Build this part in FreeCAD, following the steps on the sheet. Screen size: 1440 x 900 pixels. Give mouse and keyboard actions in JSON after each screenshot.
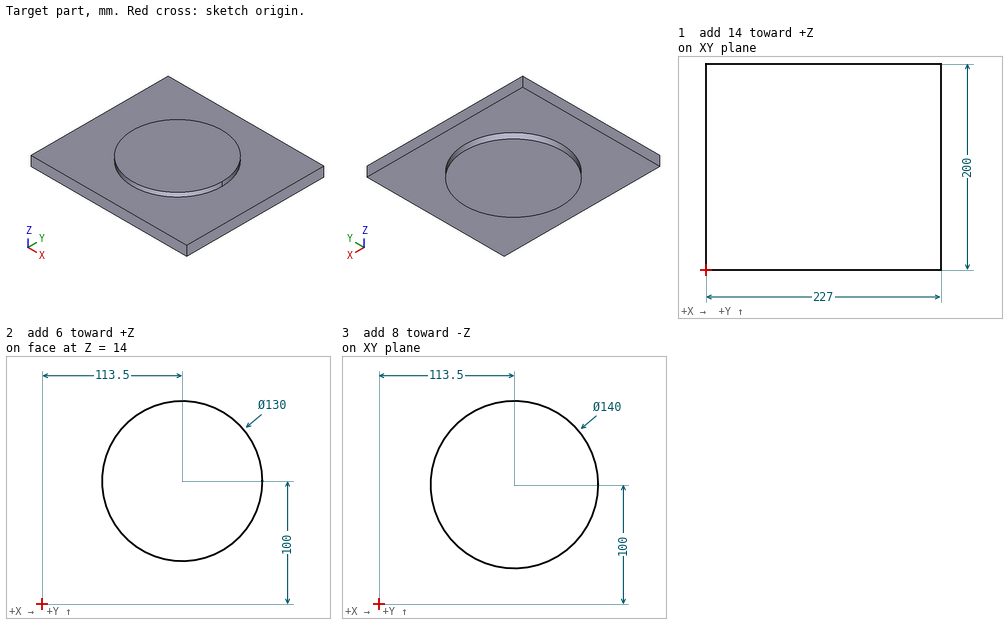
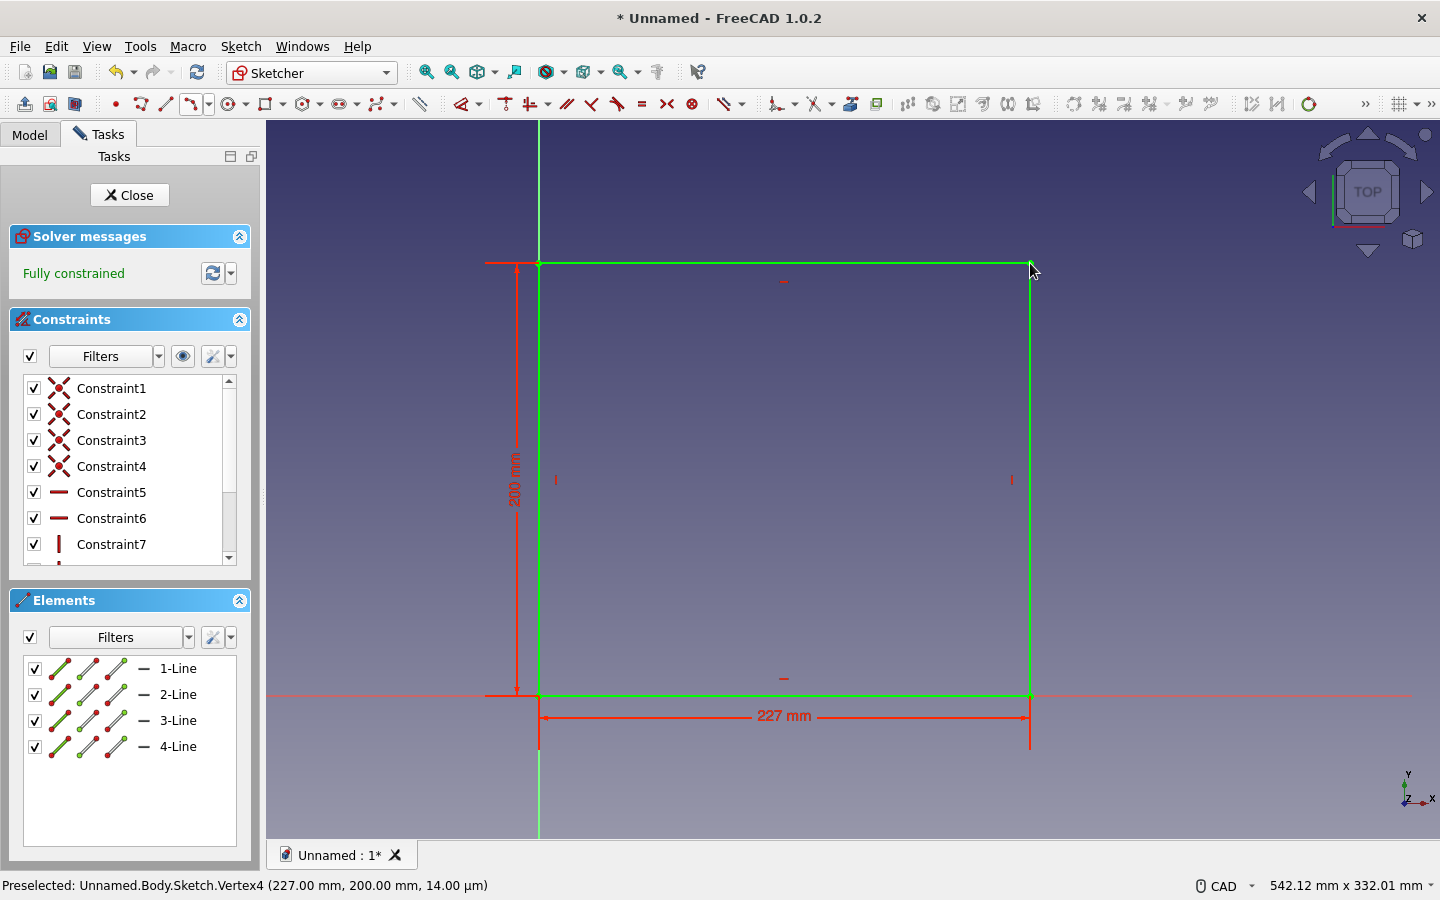
{"action": "left_click", "coordinate": [130, 195]}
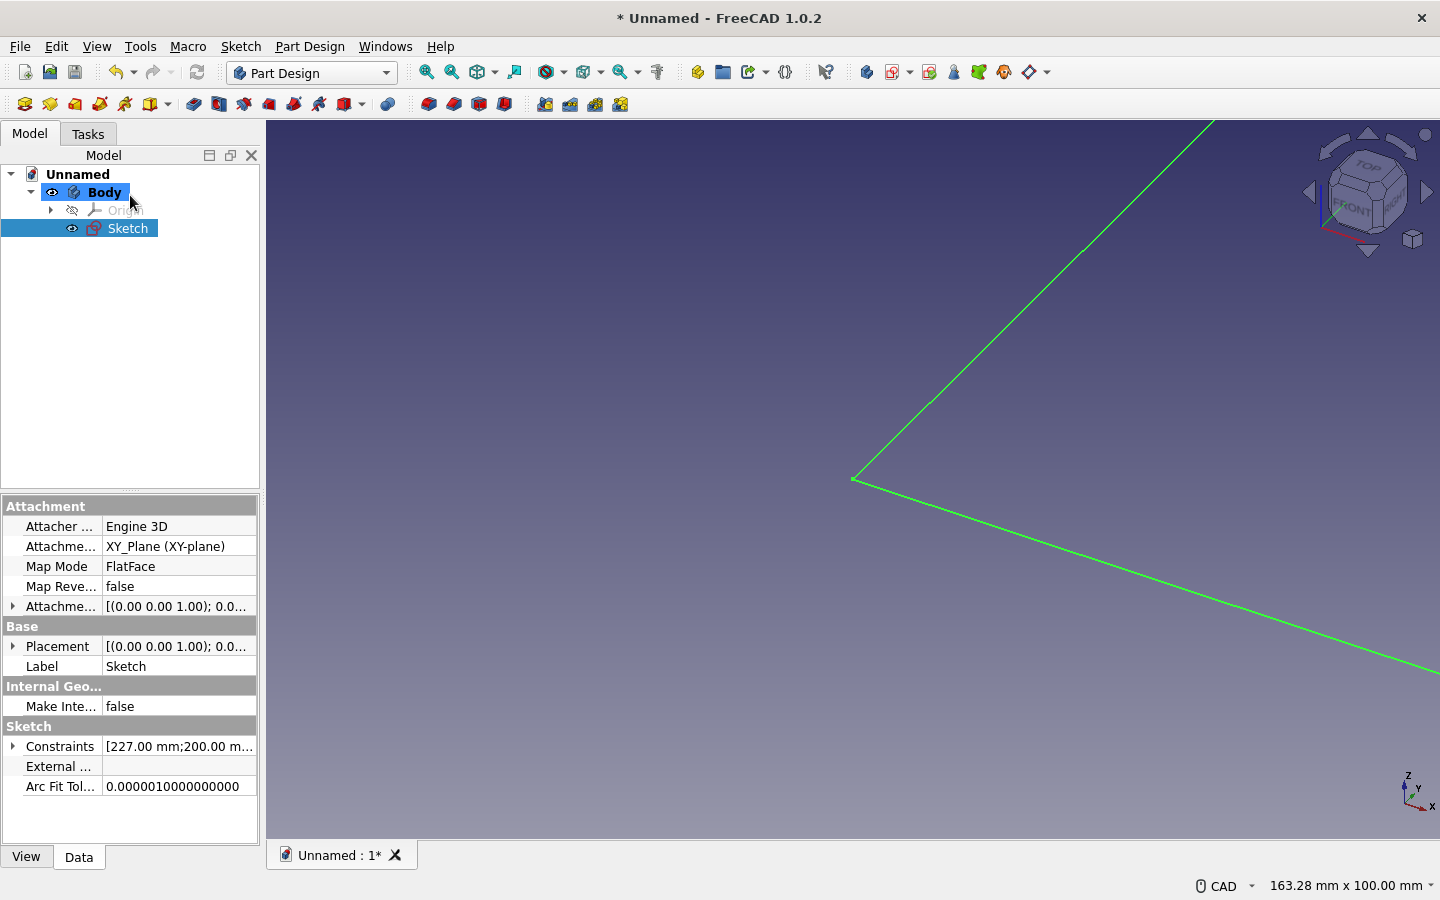
{"action": "left_click", "coordinate": [25, 104]}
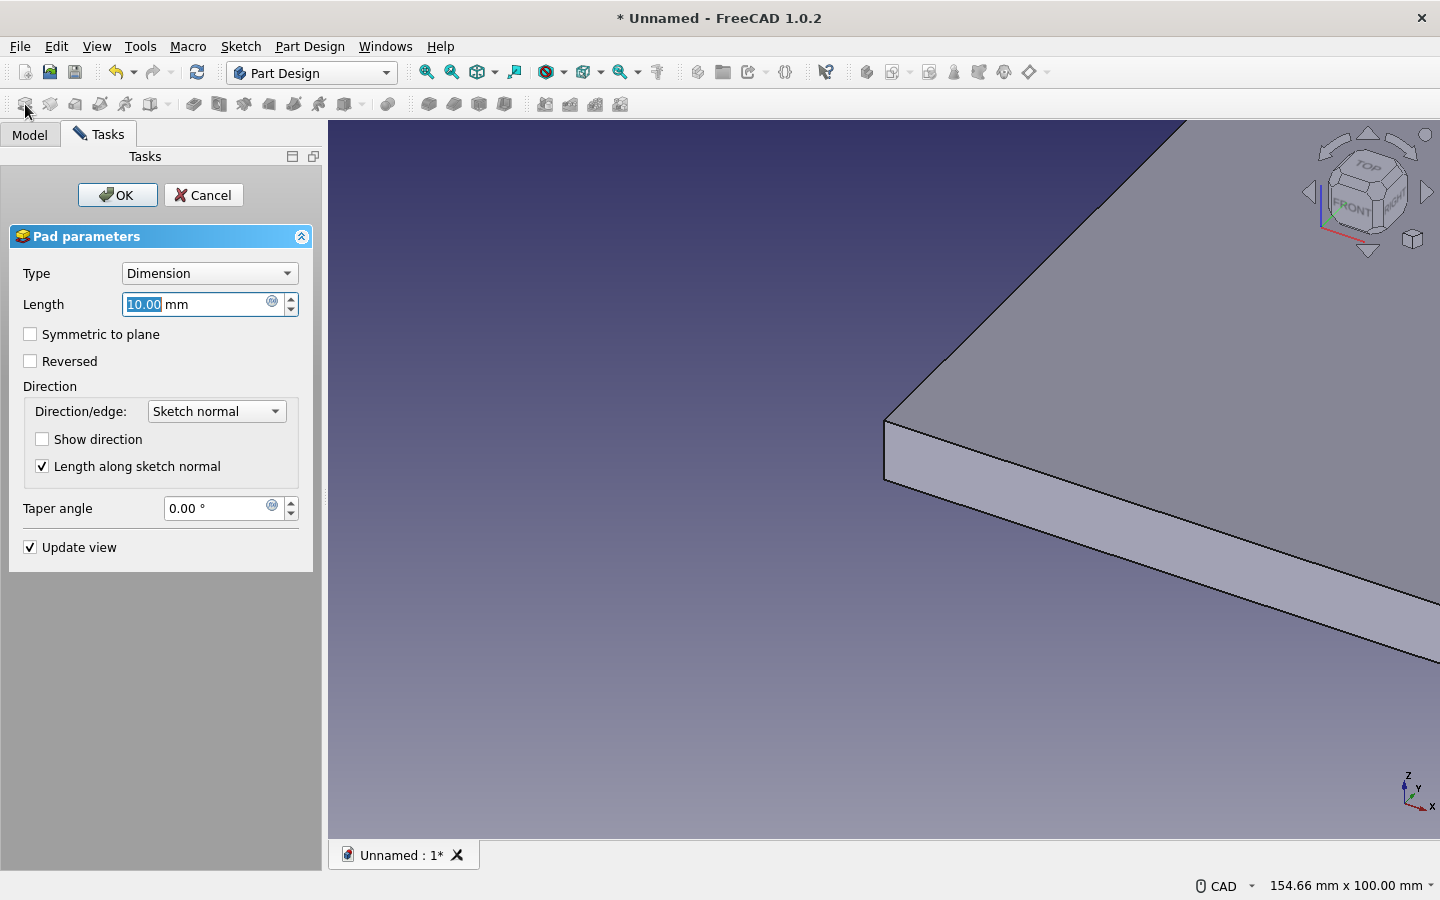
{"action": "type", "text": "14"}
{"action": "key", "text": "Tab"}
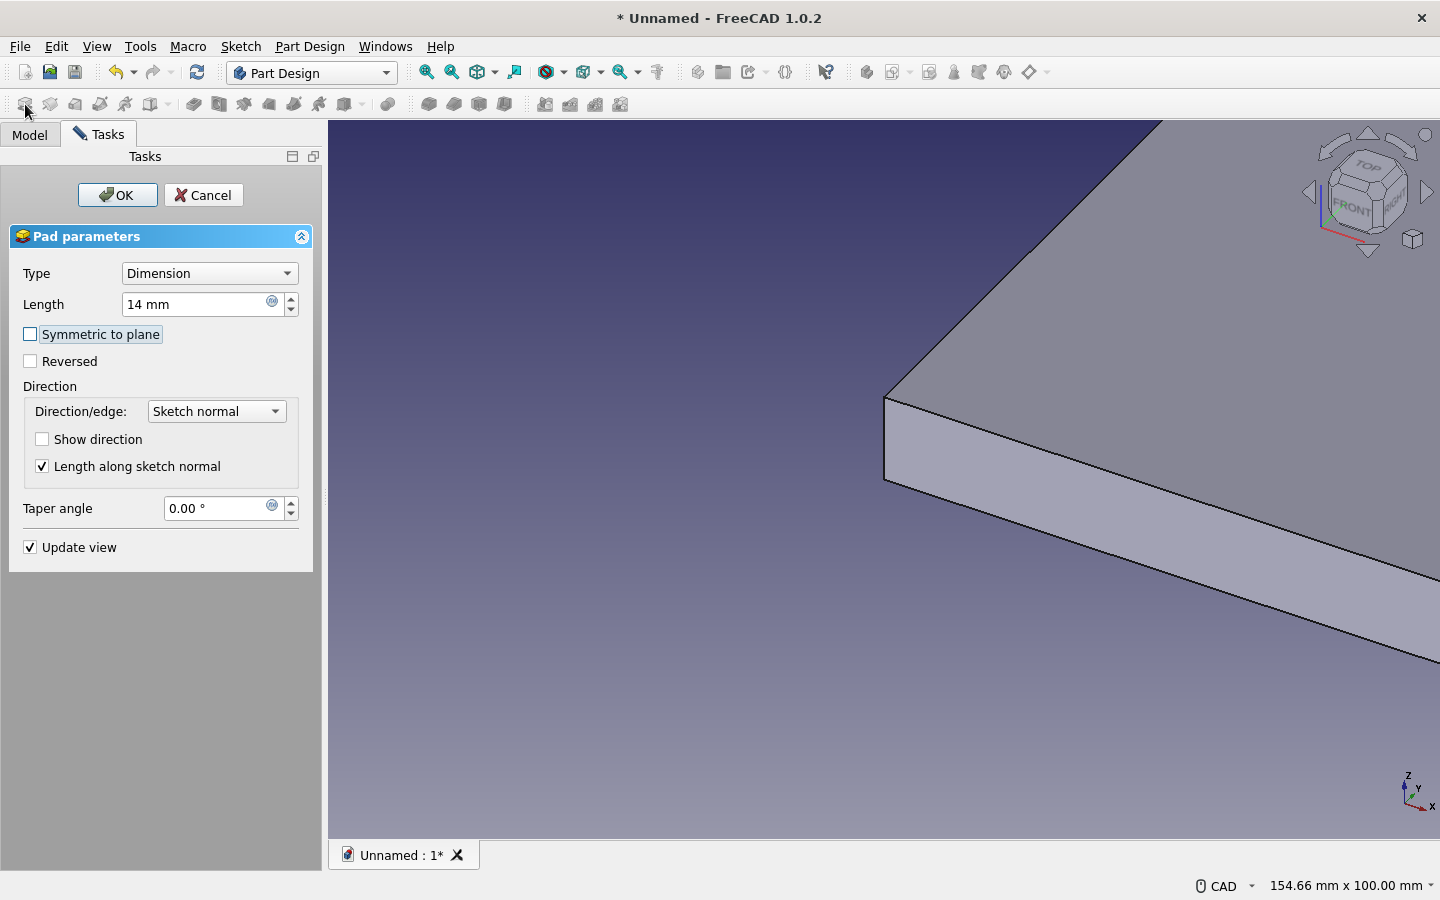
{"action": "left_click", "coordinate": [118, 195]}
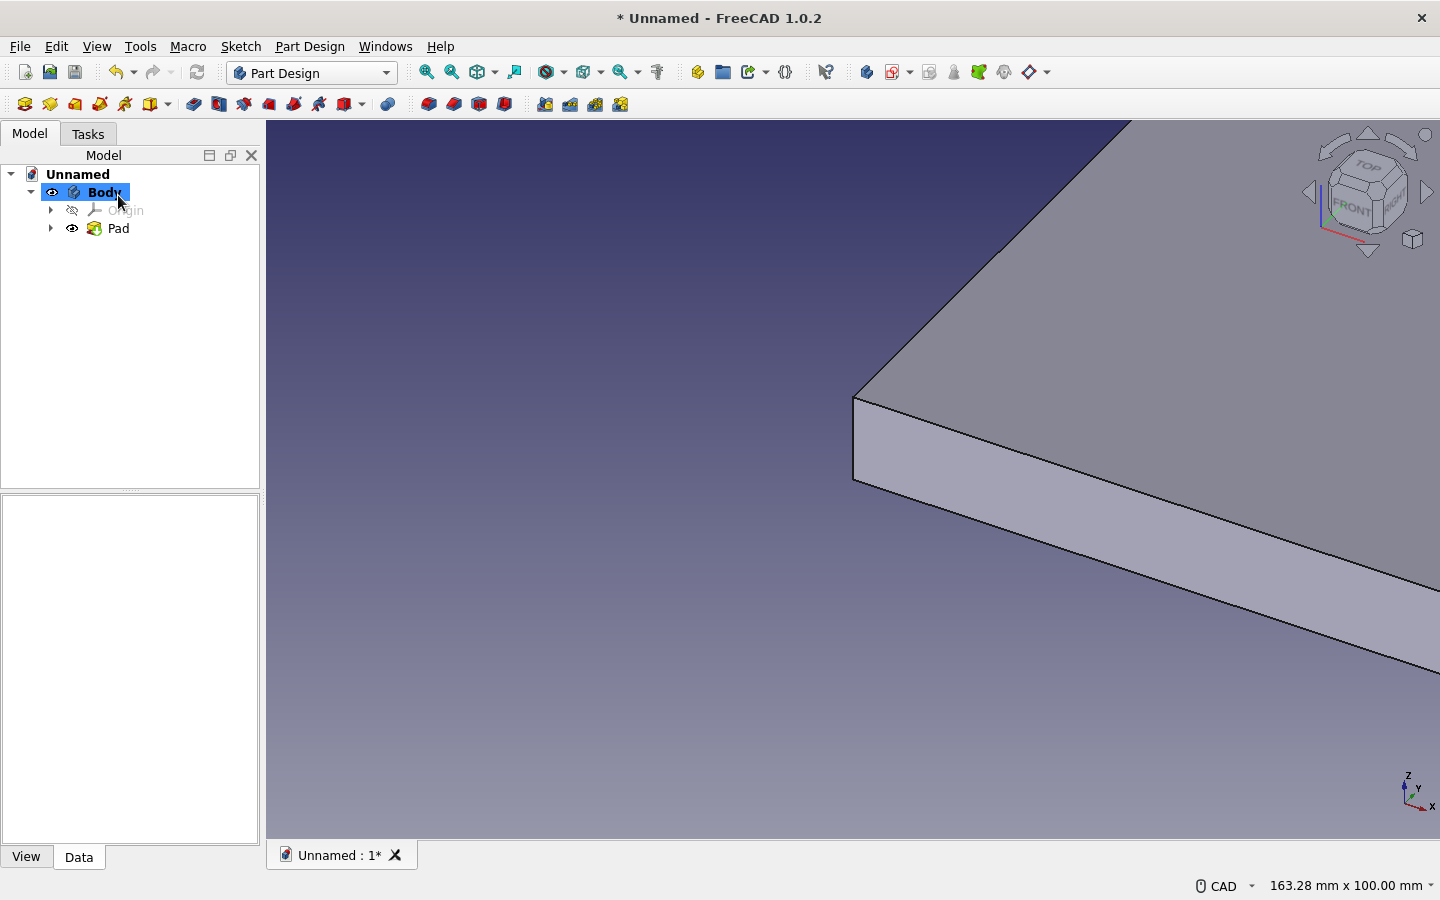
{"action": "left_click", "coordinate": [427, 72]}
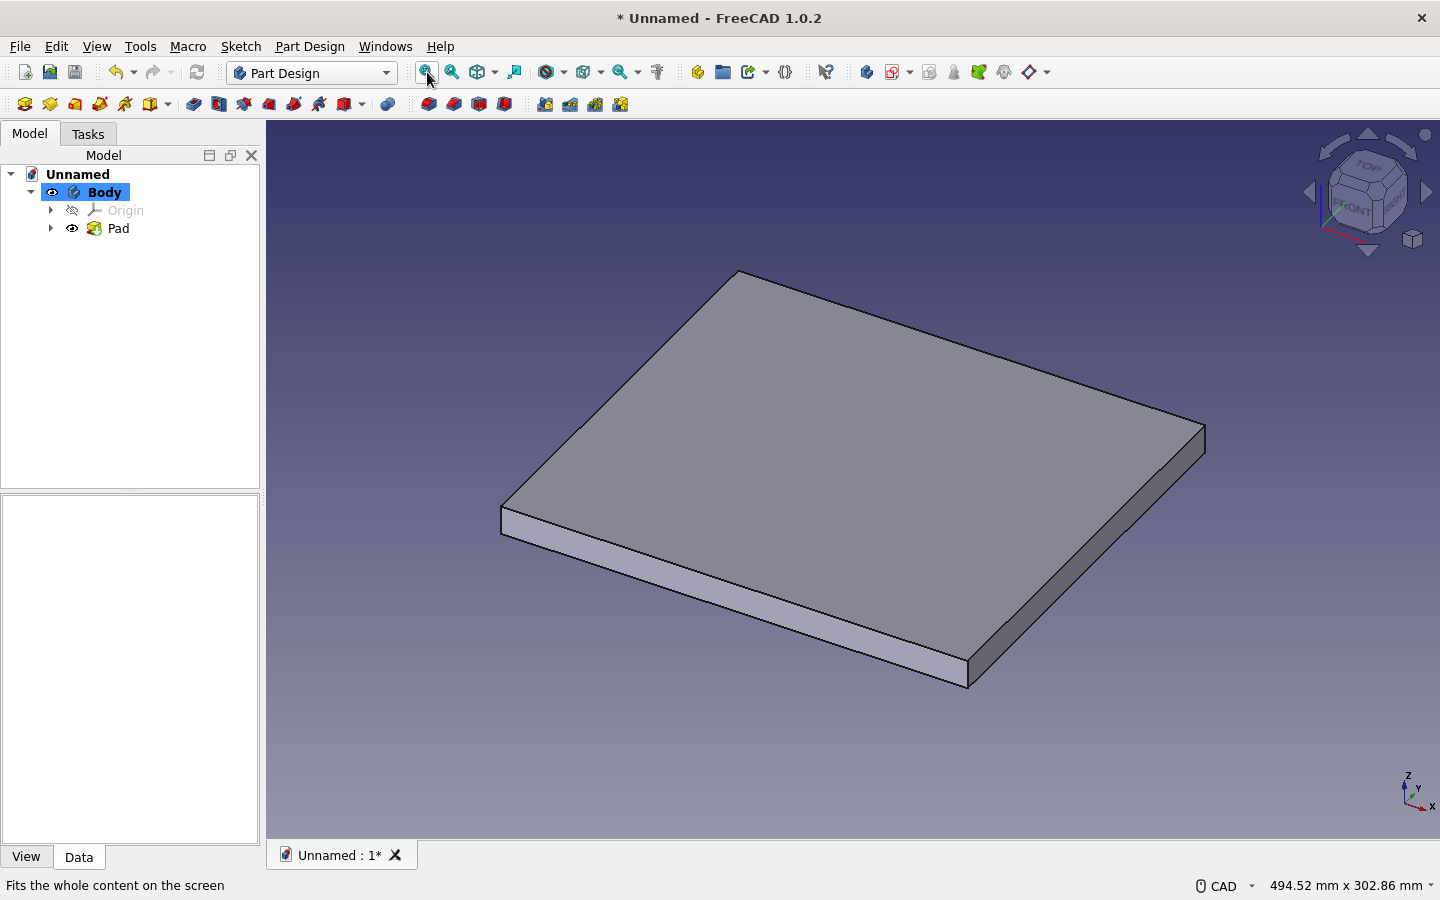
{"action": "left_click", "coordinate": [853, 465]}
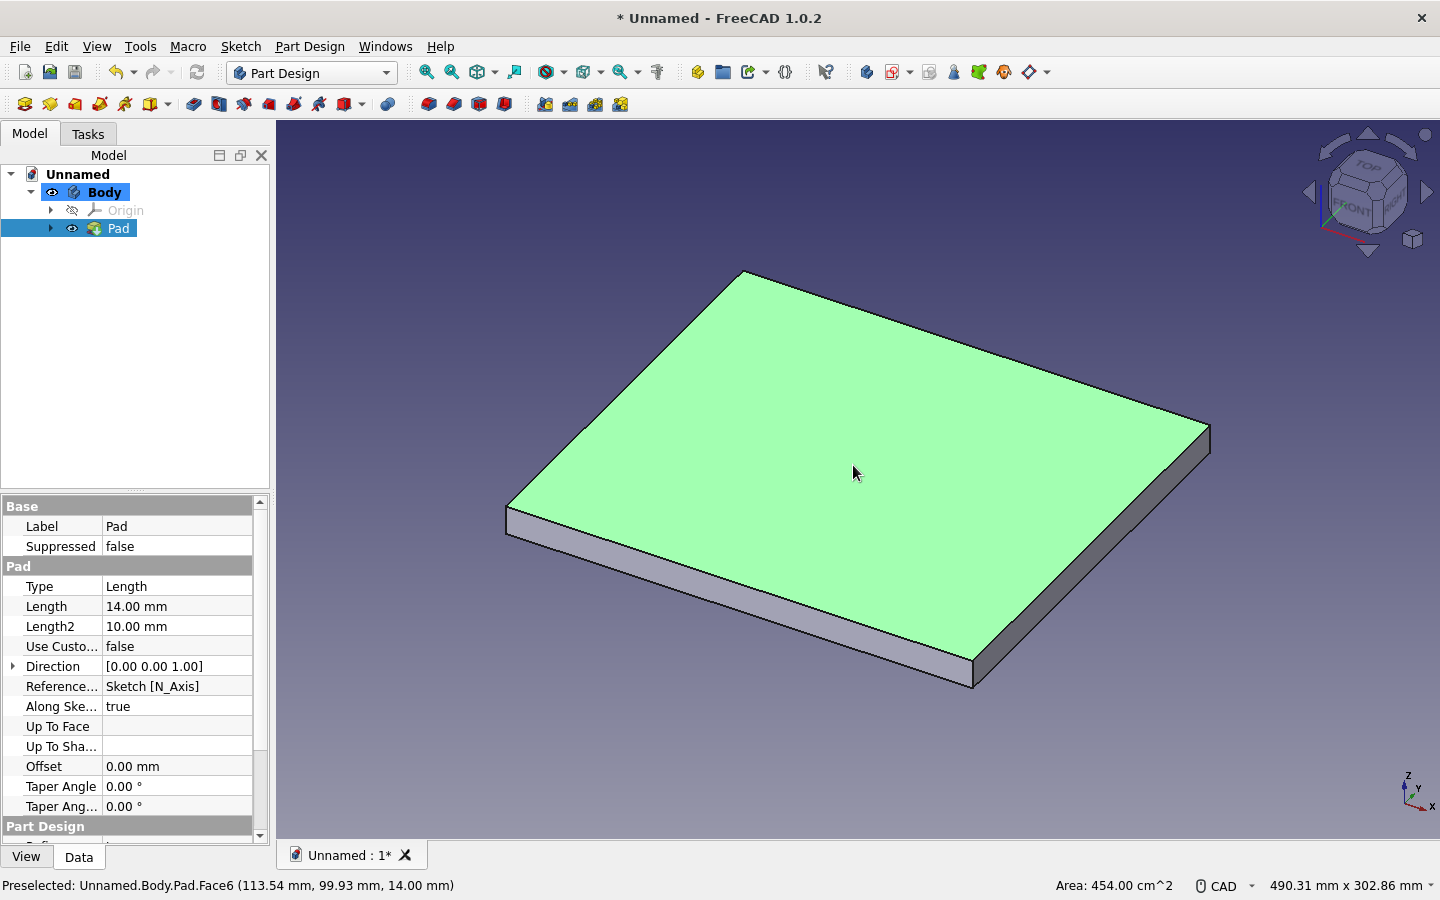
{"action": "left_click", "coordinate": [892, 72]}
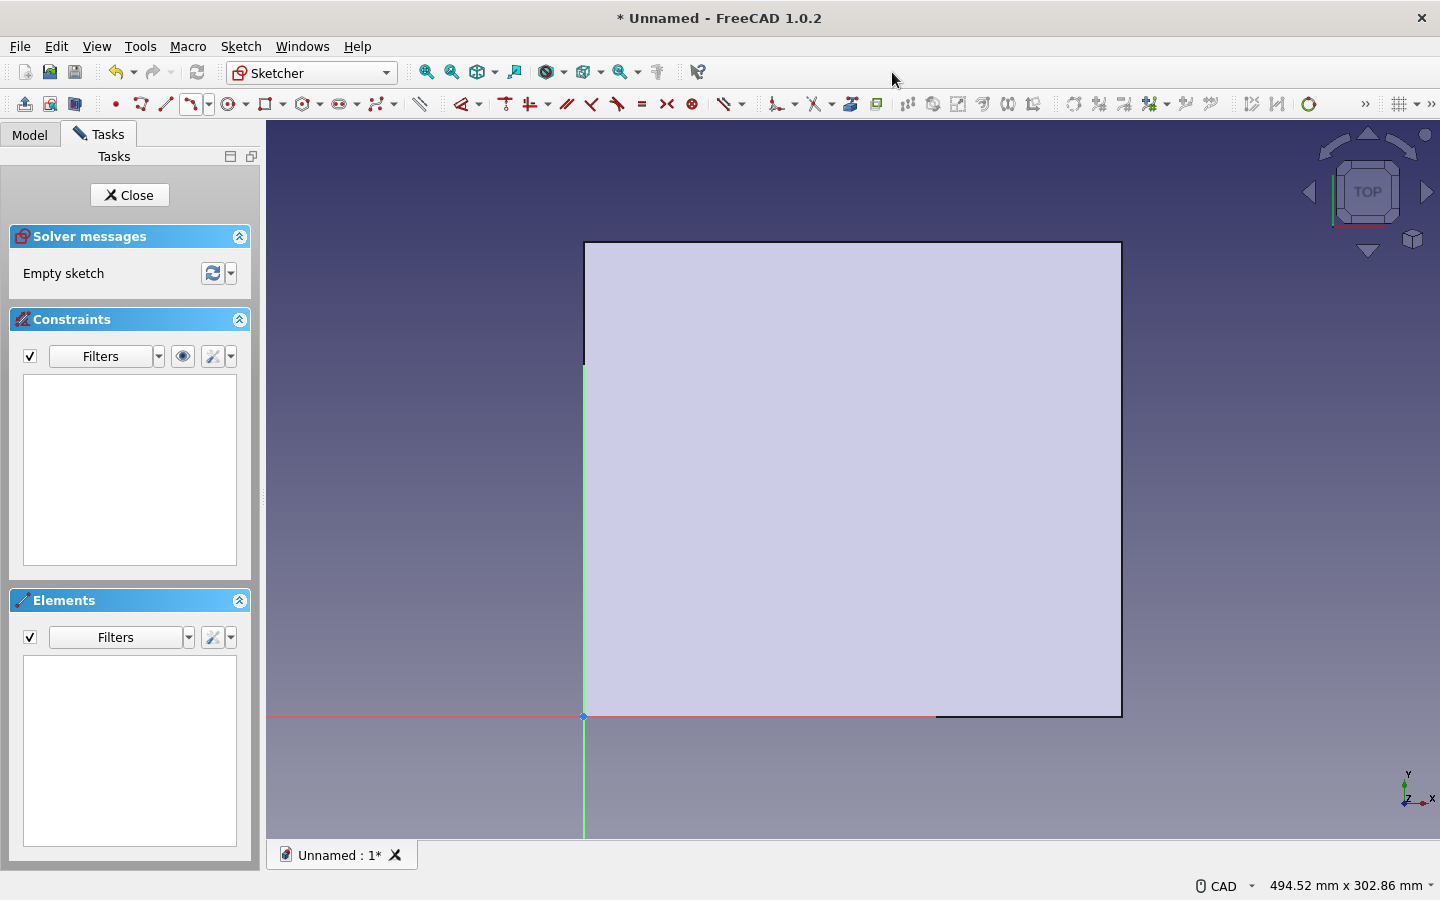
{"action": "key", "text": "g c"}